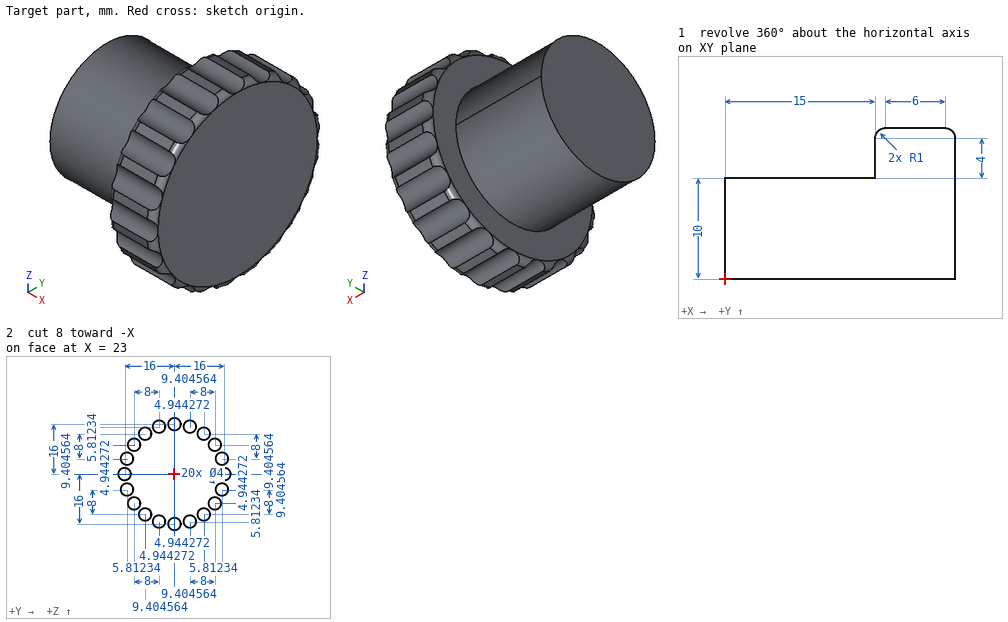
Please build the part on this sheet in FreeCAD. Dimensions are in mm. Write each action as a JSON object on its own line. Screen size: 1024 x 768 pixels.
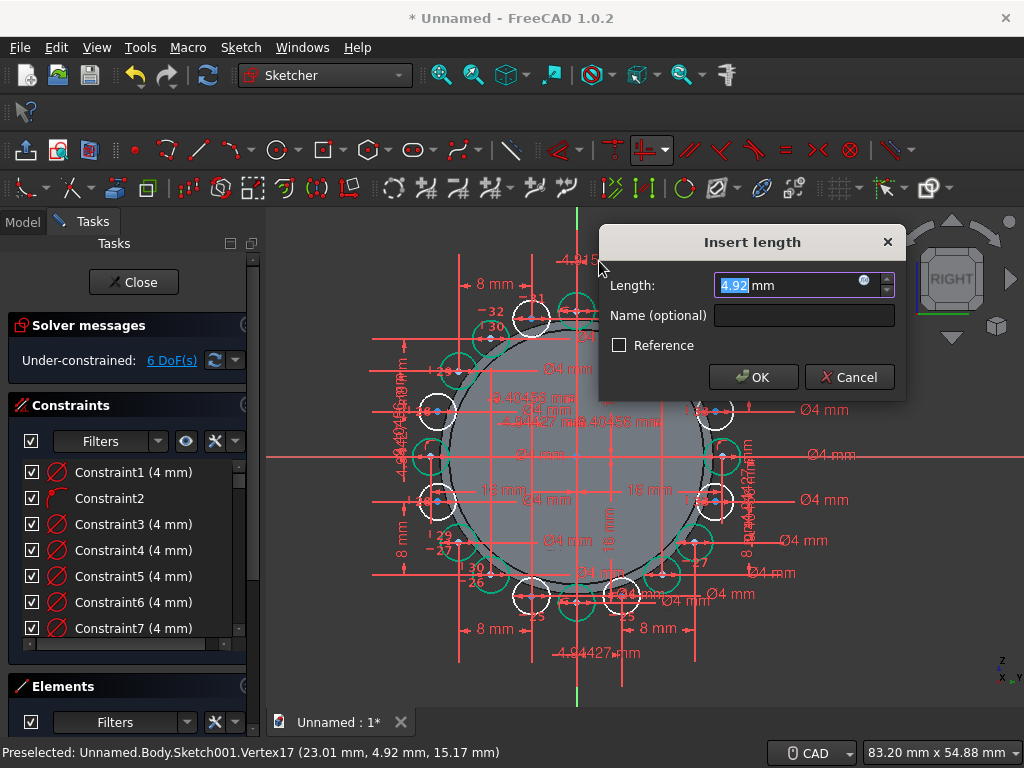
{"action": "type", "text": "4.944272"}
{"action": "key", "text": "Return"}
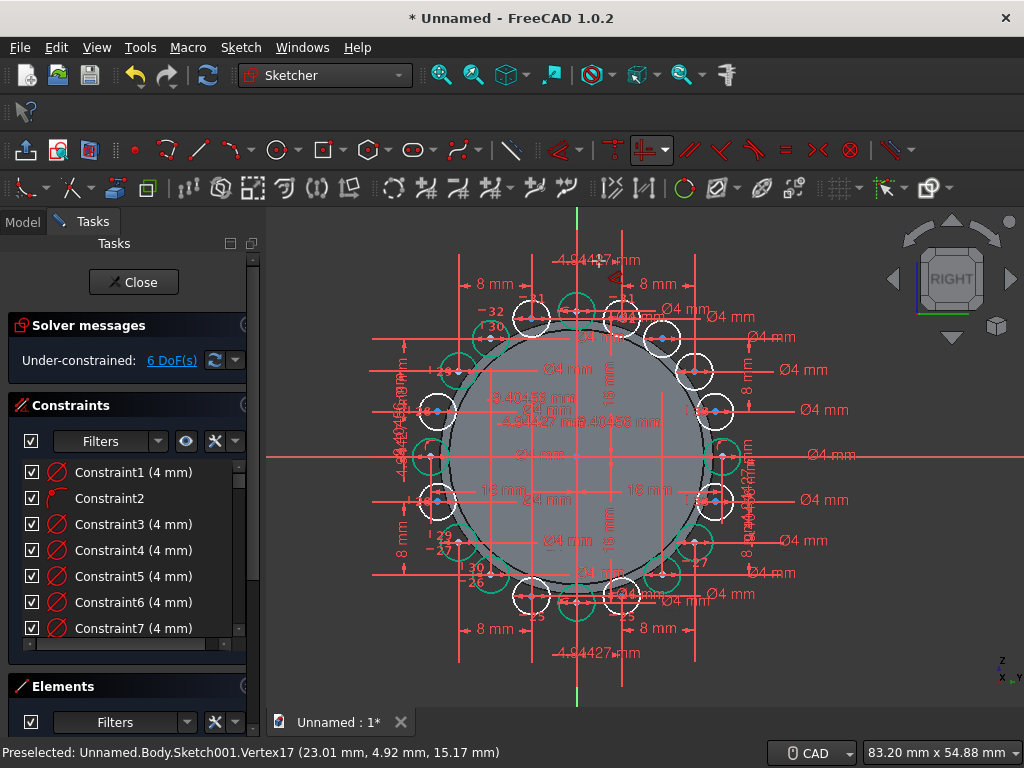
{"action": "left_click", "coordinate": [662, 339]}
{"action": "left_click", "coordinate": [619, 563]}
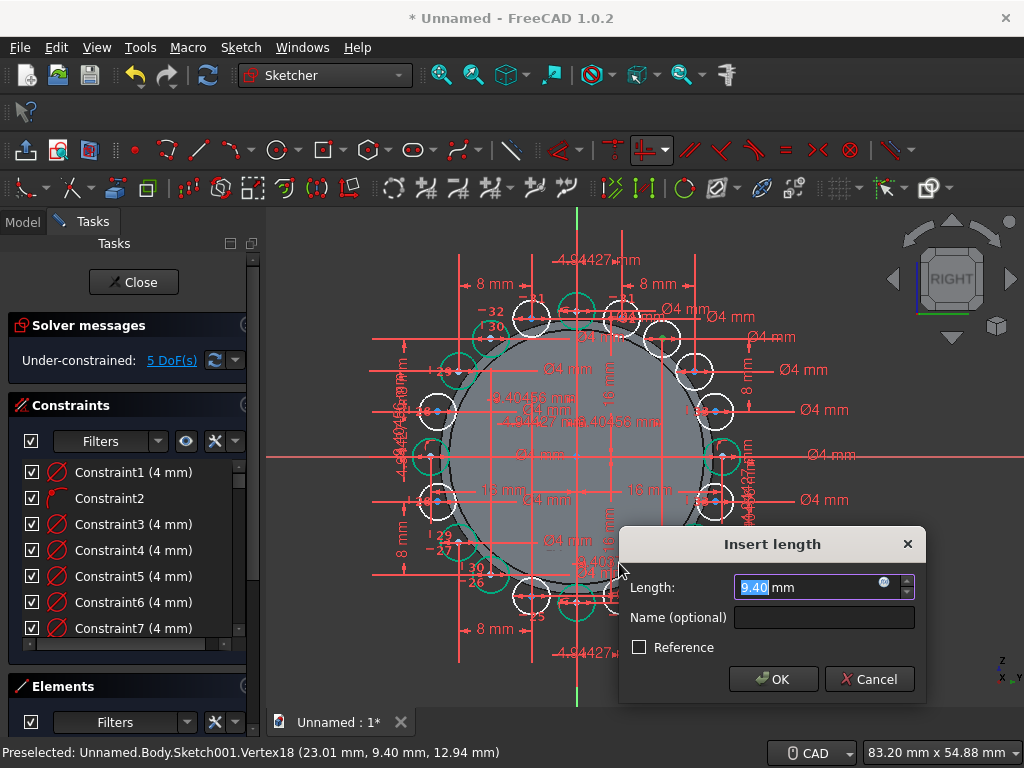
{"action": "type", "text": "9.404564"}
{"action": "key", "text": "Return"}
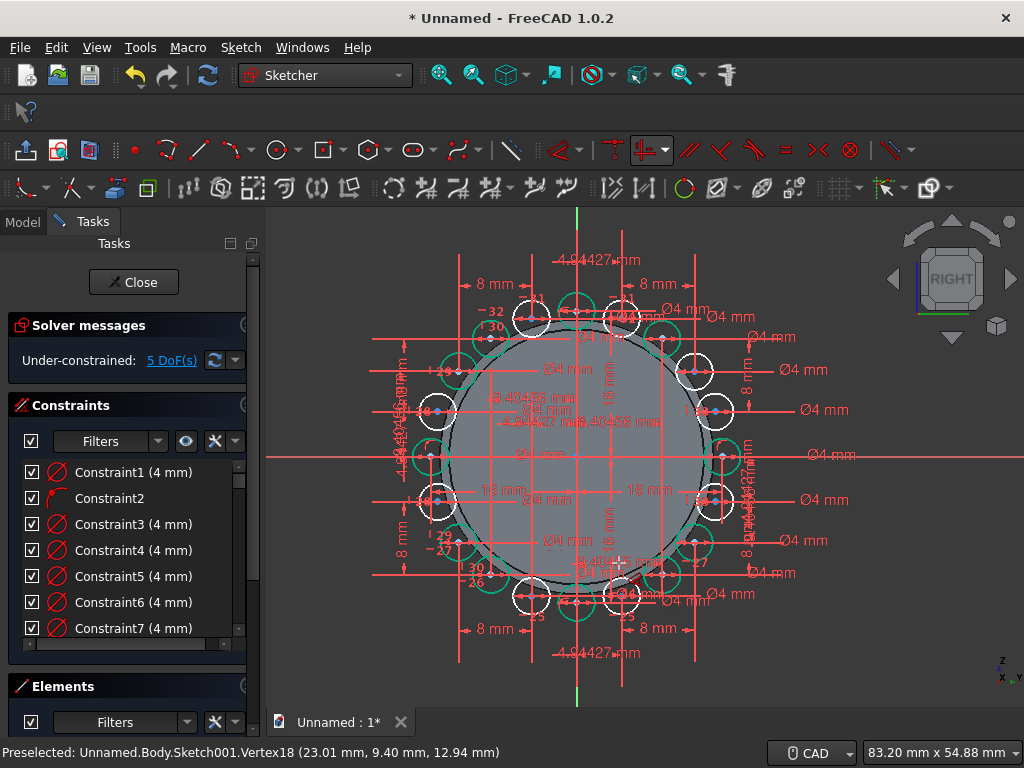
{"action": "left_click", "coordinate": [695, 372]}
{"action": "left_click", "coordinate": [753, 414]}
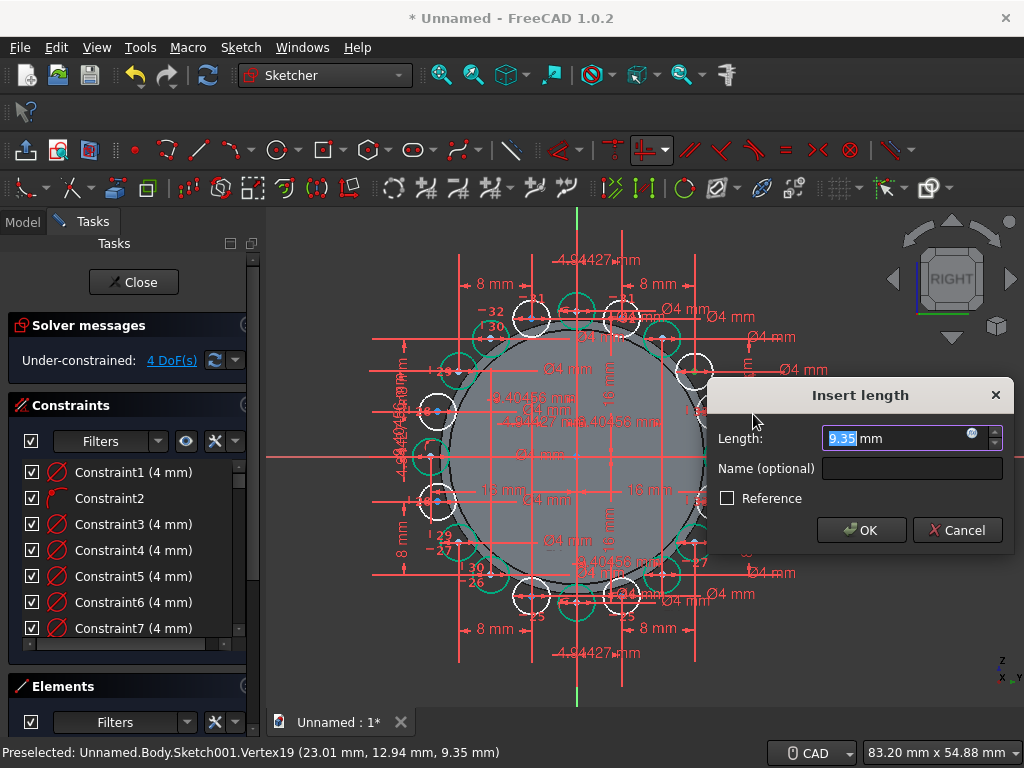
{"action": "type", "text": "9.404564"}
{"action": "key", "text": "Return"}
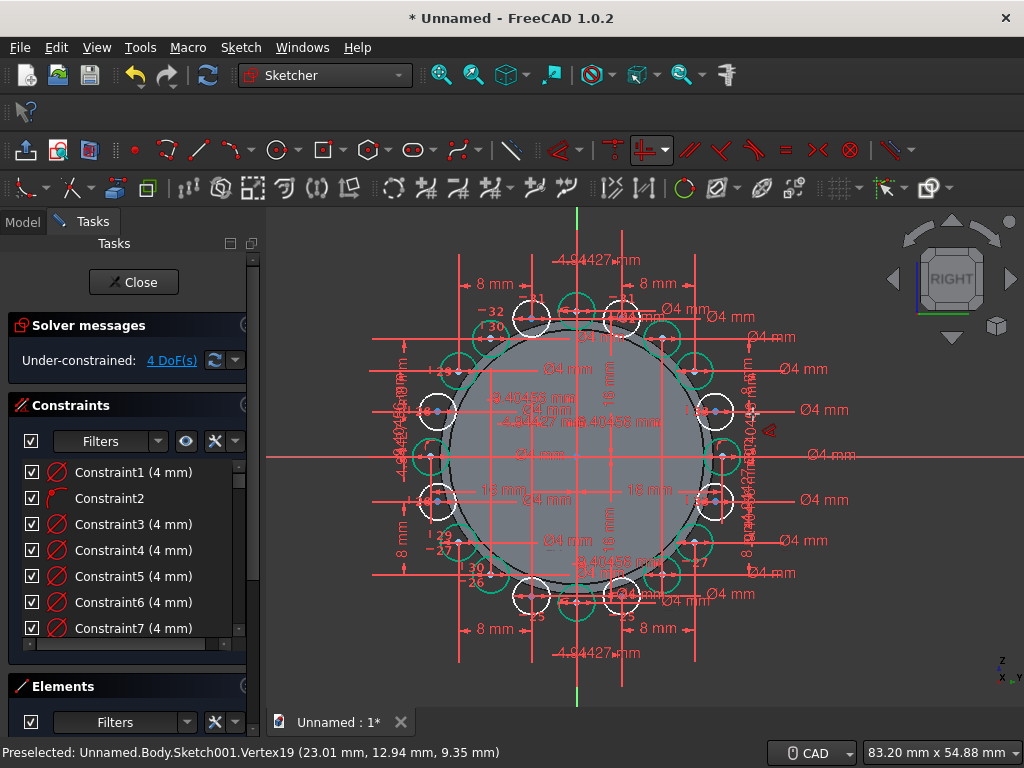
{"action": "left_click", "coordinate": [715, 502]}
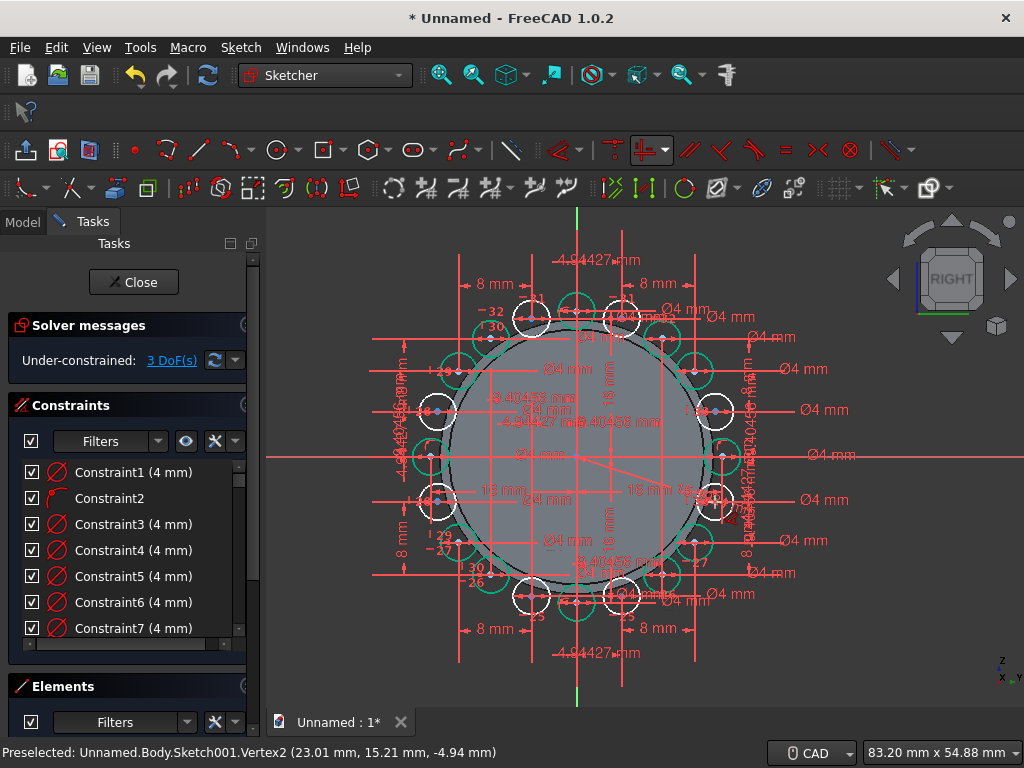
{"action": "left_click", "coordinate": [662, 575]}
{"action": "left_click", "coordinate": [689, 609]}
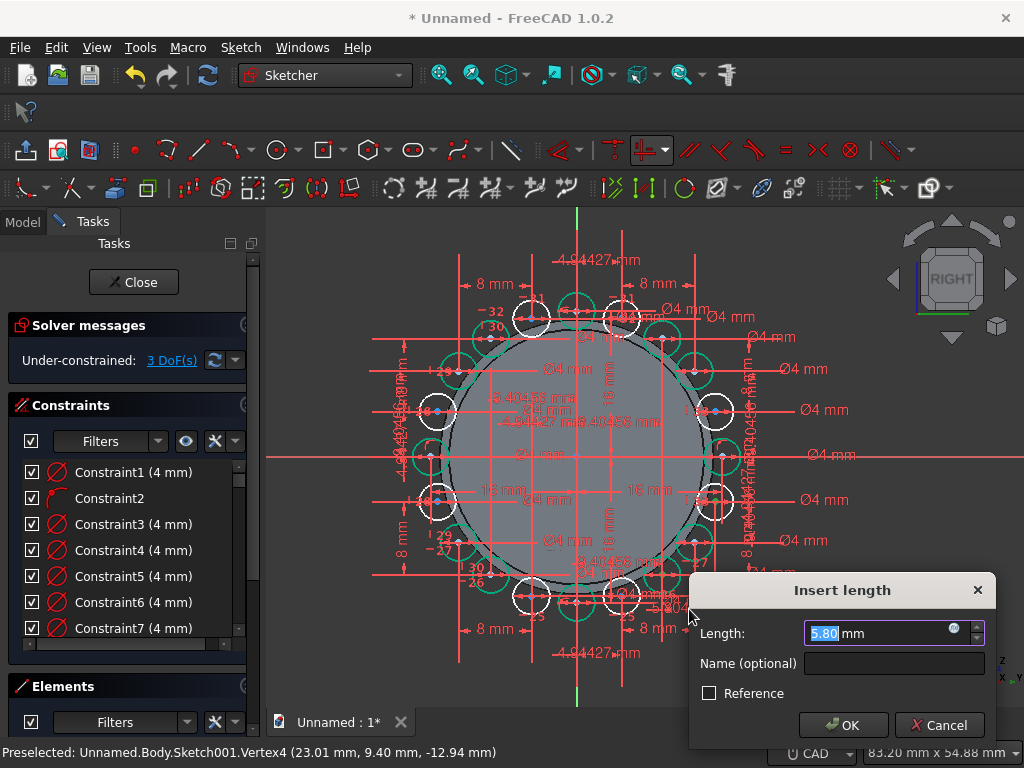
{"action": "type", "text": "5.81234"}
{"action": "key", "text": "Return"}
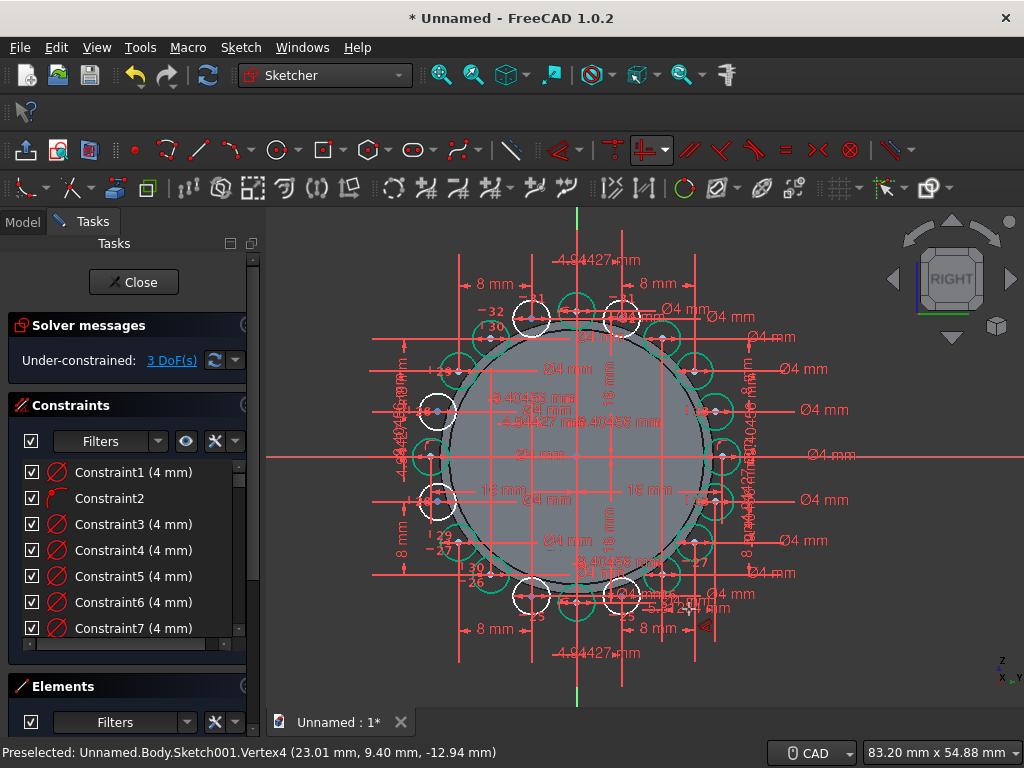
{"action": "left_click", "coordinate": [695, 543]}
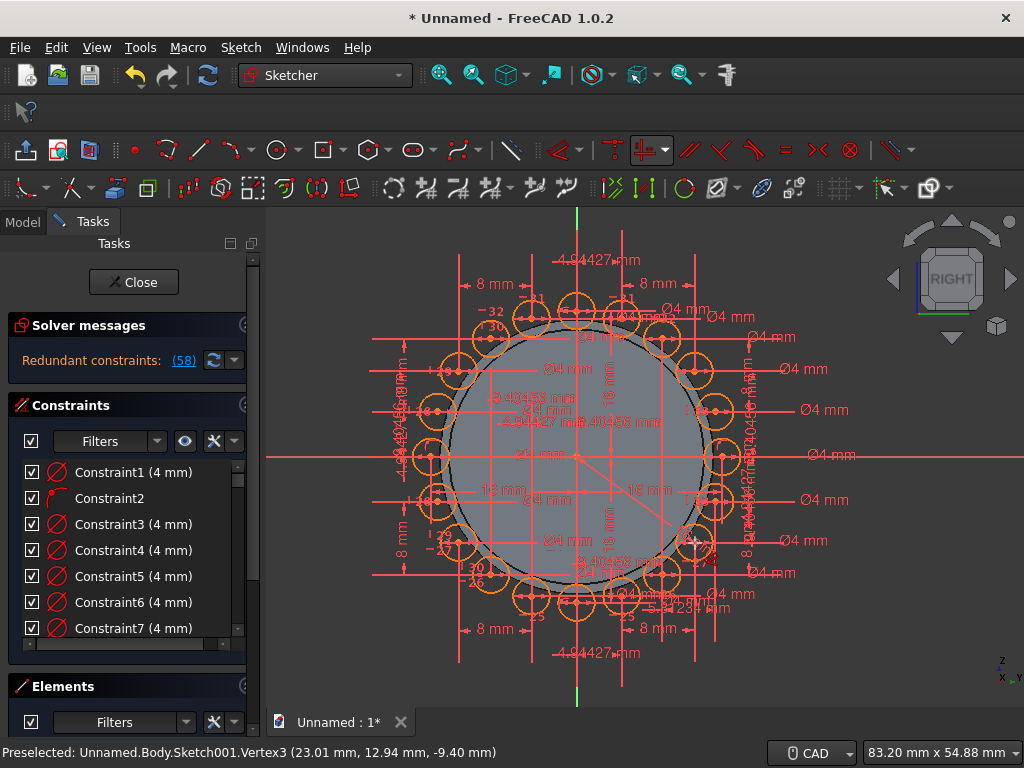
{"action": "left_click", "coordinate": [622, 596]}
{"action": "left_click", "coordinate": [729, 569]}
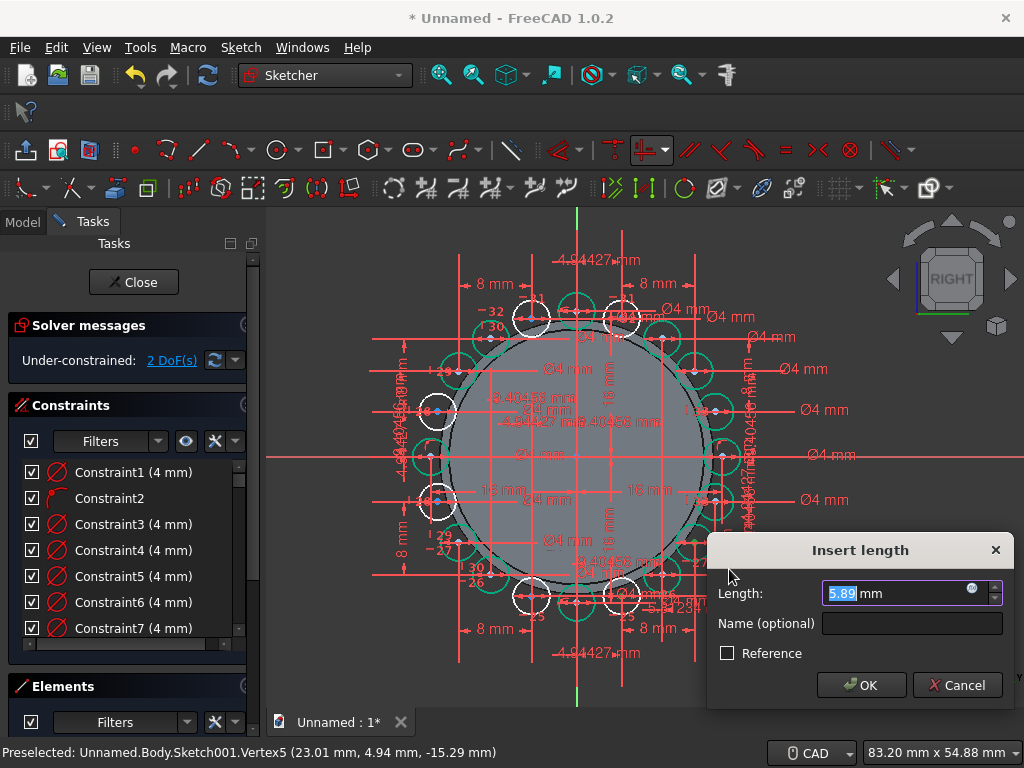
{"action": "type", "text": "5.81234"}
{"action": "key", "text": "Return"}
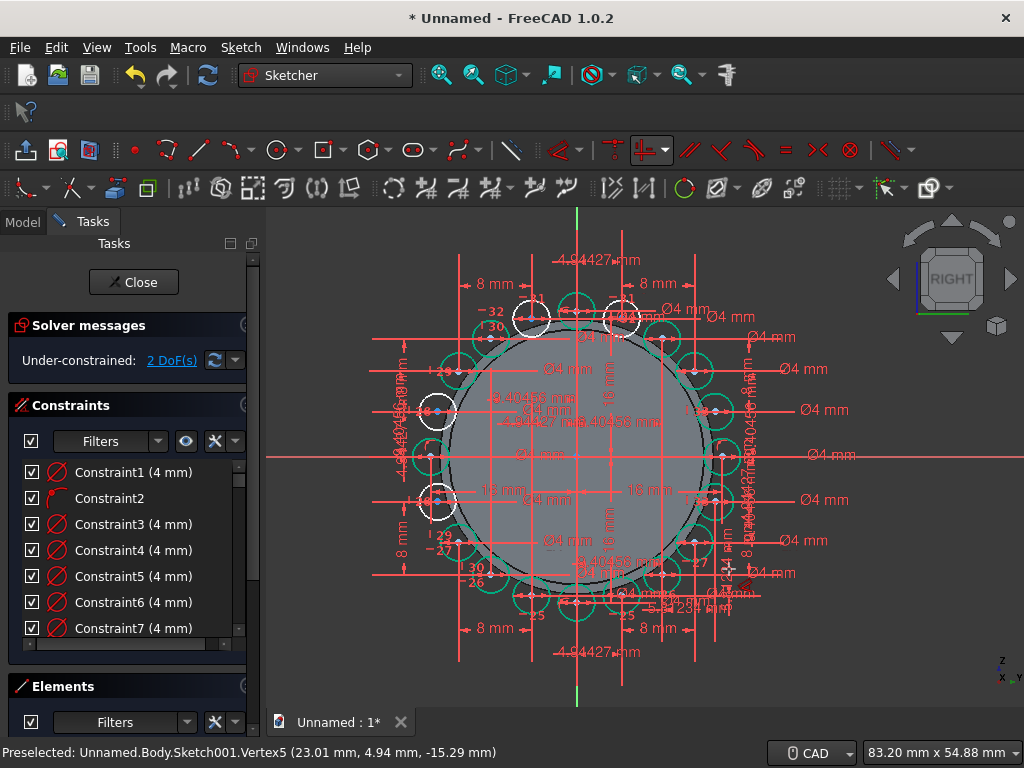
{"action": "left_click", "coordinate": [491, 575]}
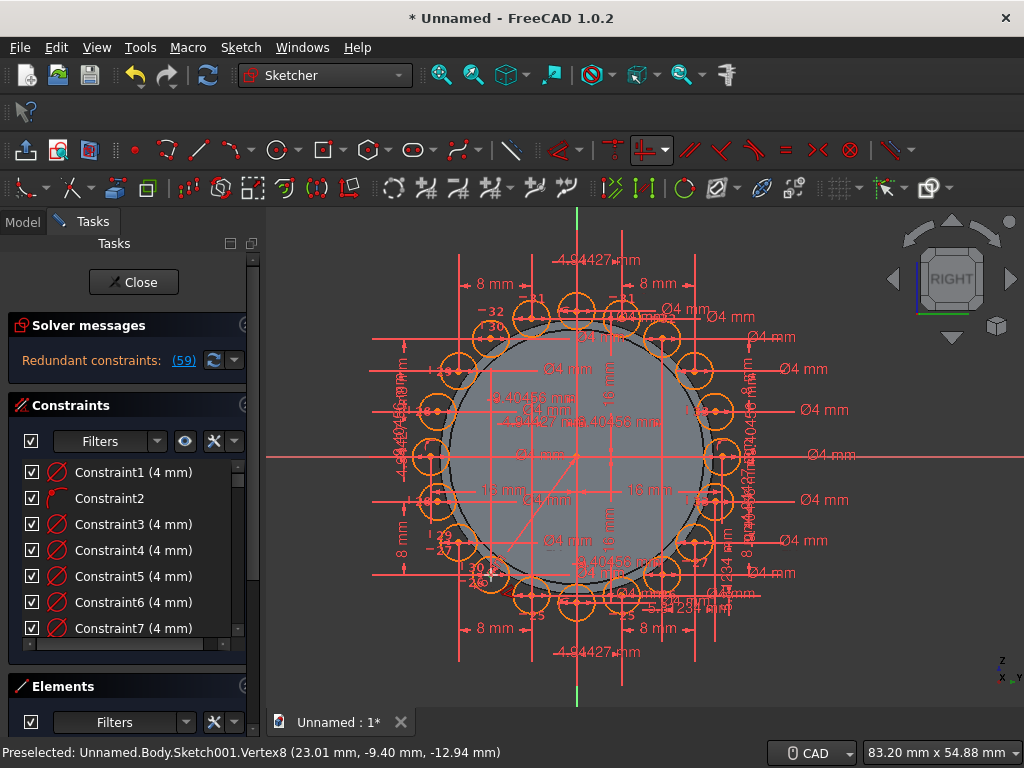
{"action": "left_click", "coordinate": [438, 502]}
{"action": "left_click", "coordinate": [464, 609]}